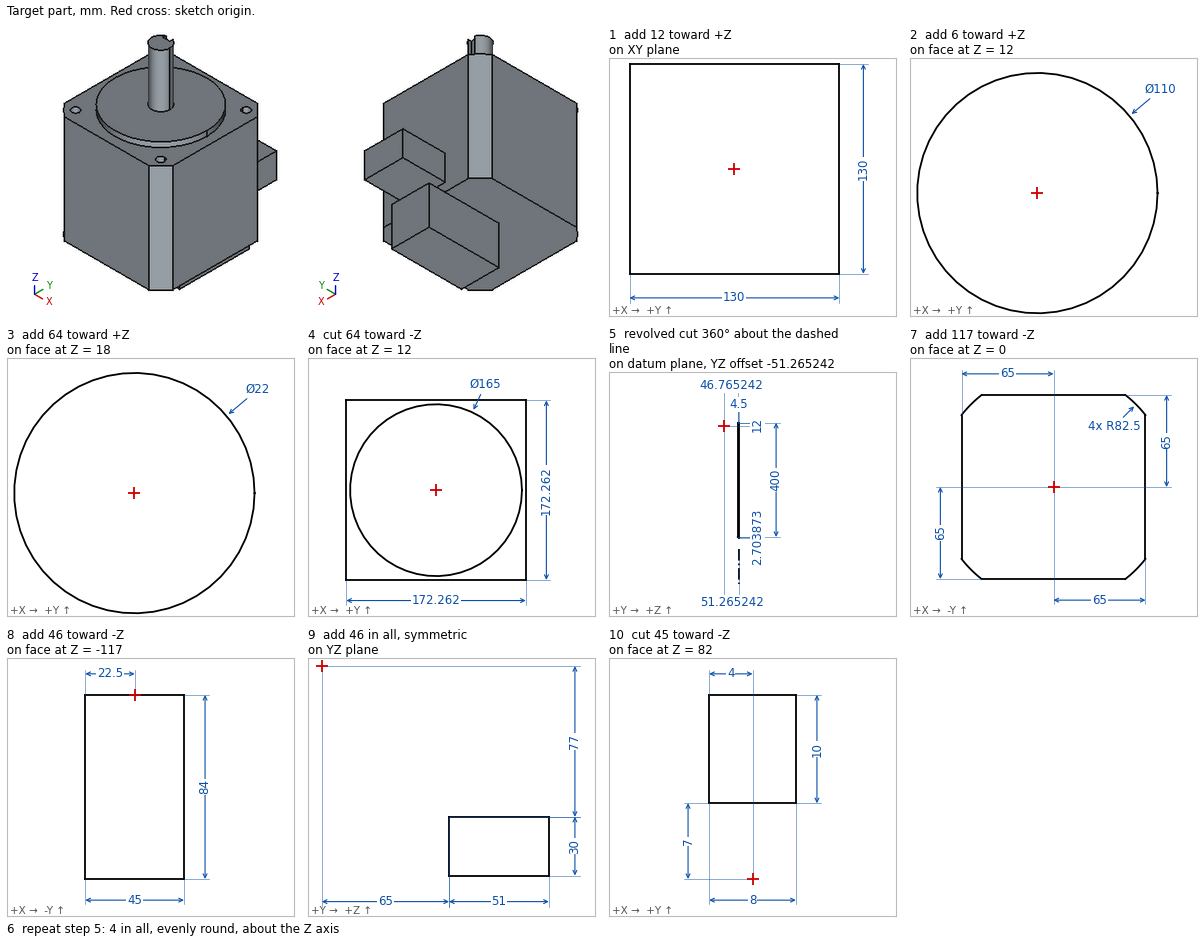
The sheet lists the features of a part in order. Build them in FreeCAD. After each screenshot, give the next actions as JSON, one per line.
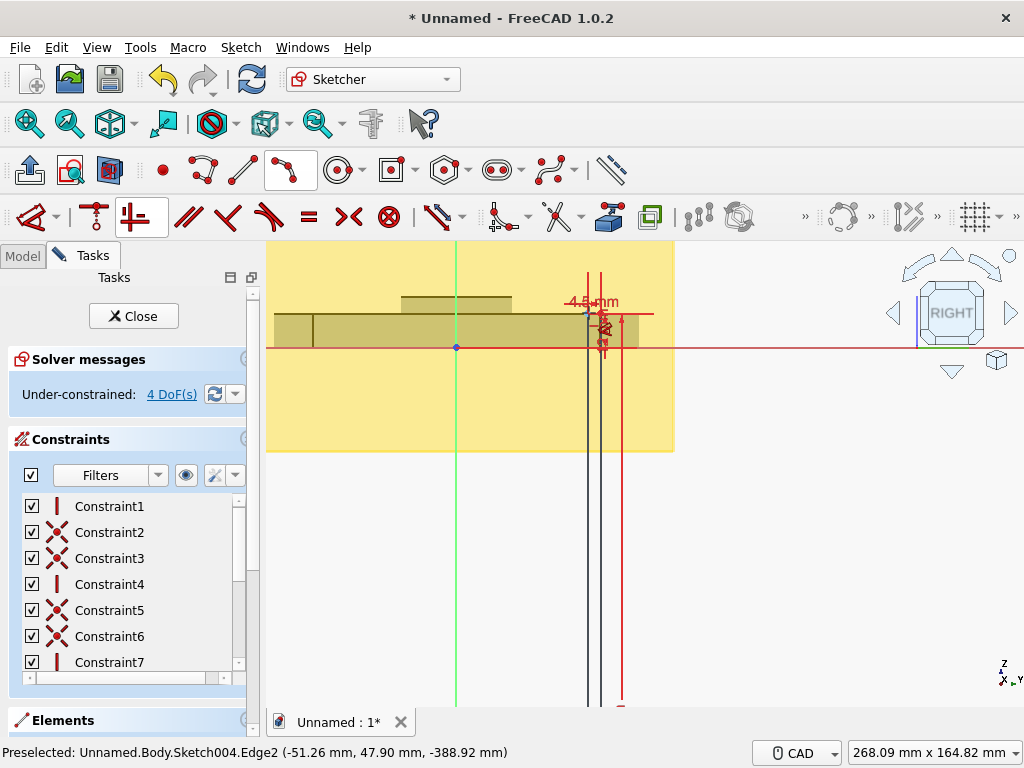
{"action": "left_click", "coordinate": [588, 314]}
{"action": "left_click", "coordinate": [522, 280]}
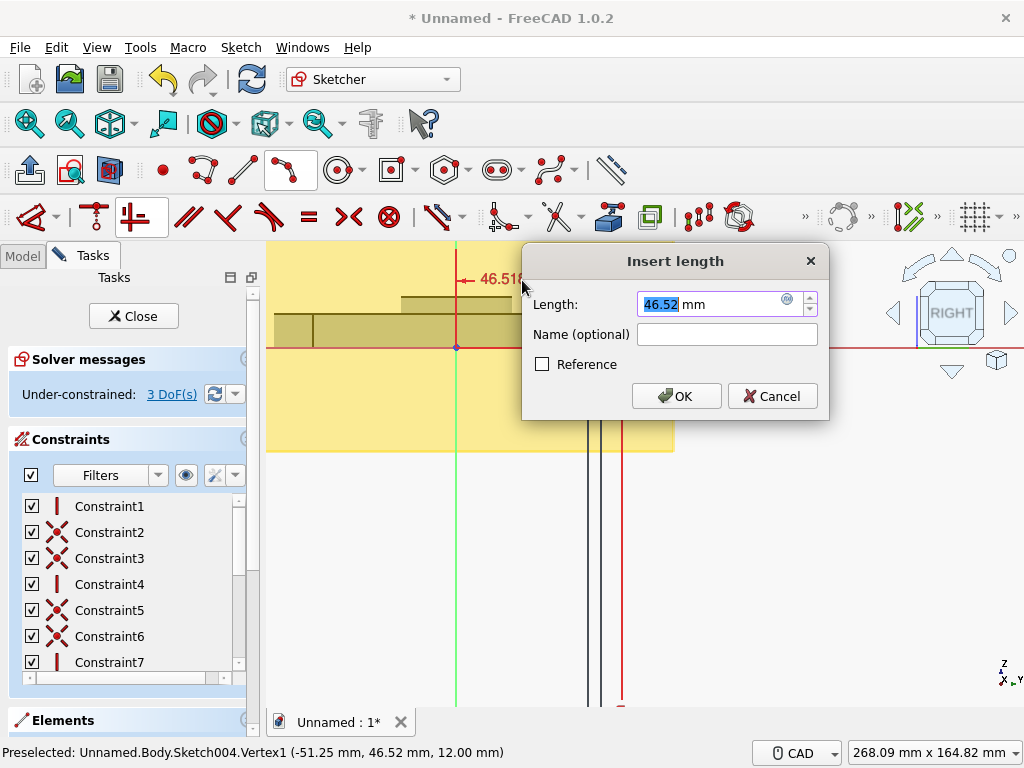
{"action": "type", "text": "46.765242"}
{"action": "key", "text": "Return"}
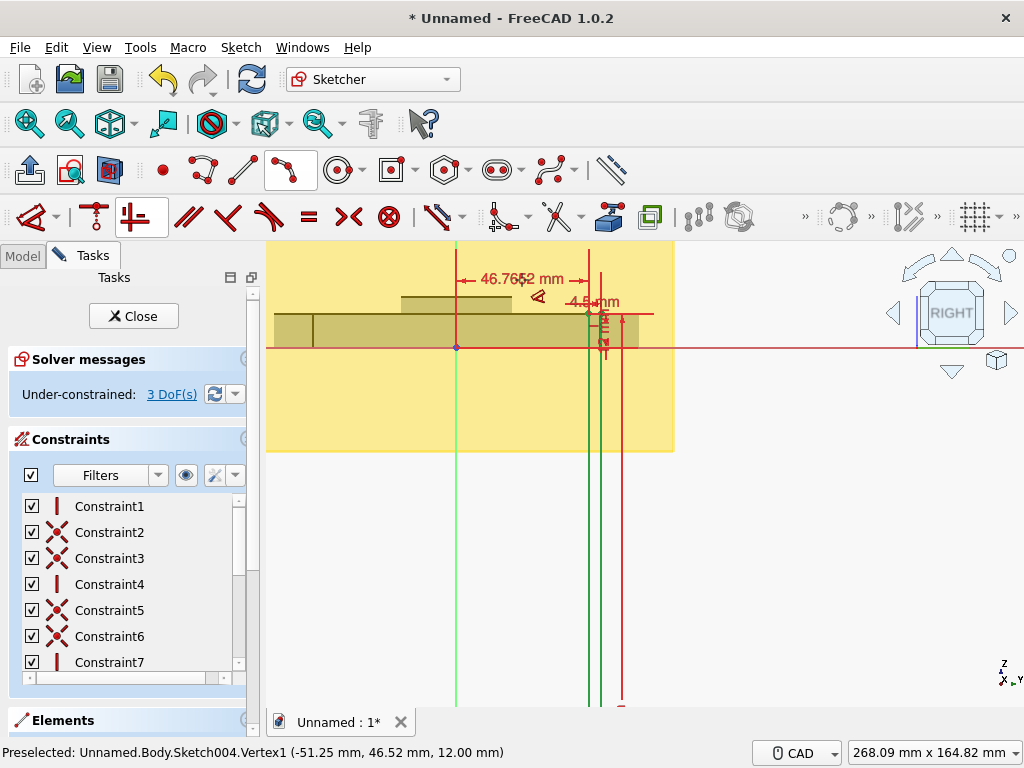
{"action": "scroll", "coordinate": [586, 348], "scroll_direction": "down", "scroll_amount": 9}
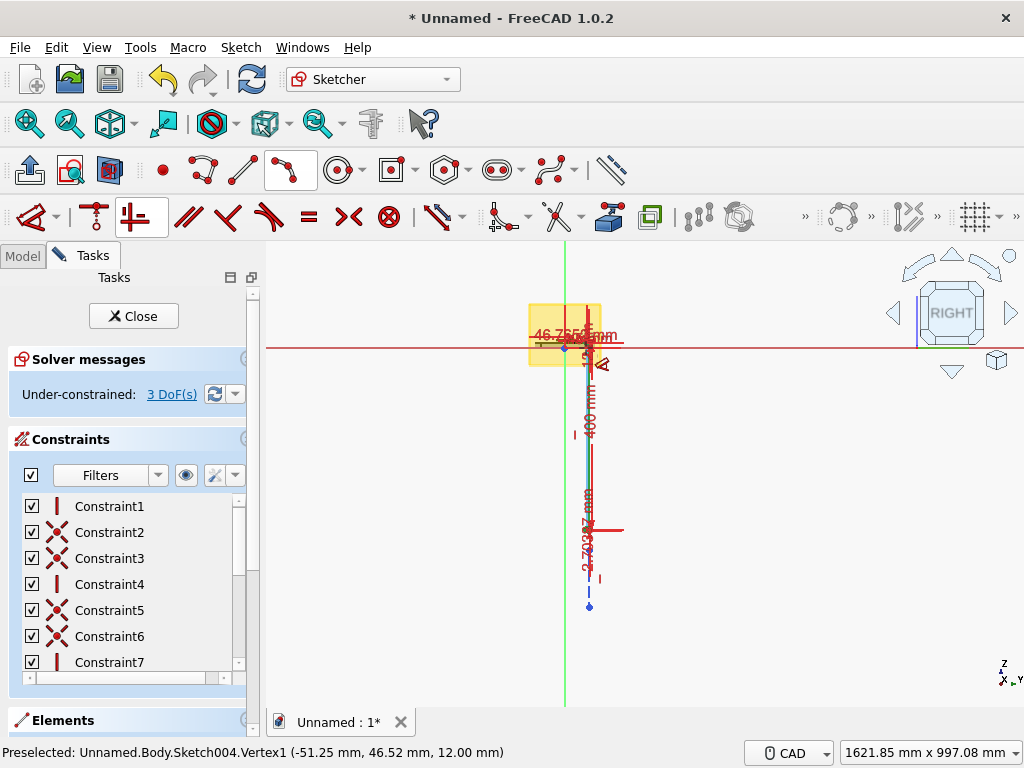
{"action": "scroll", "coordinate": [589, 550], "scroll_direction": "up", "scroll_amount": 3}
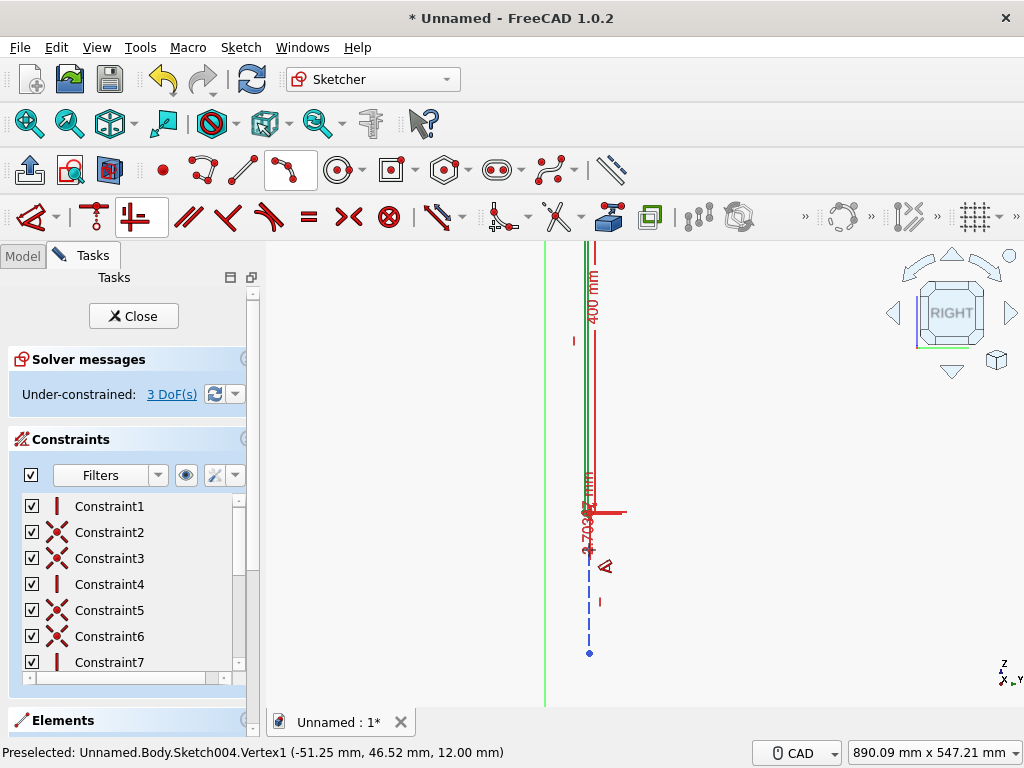
{"action": "left_click", "coordinate": [589, 550]}
{"action": "left_click", "coordinate": [567, 584]}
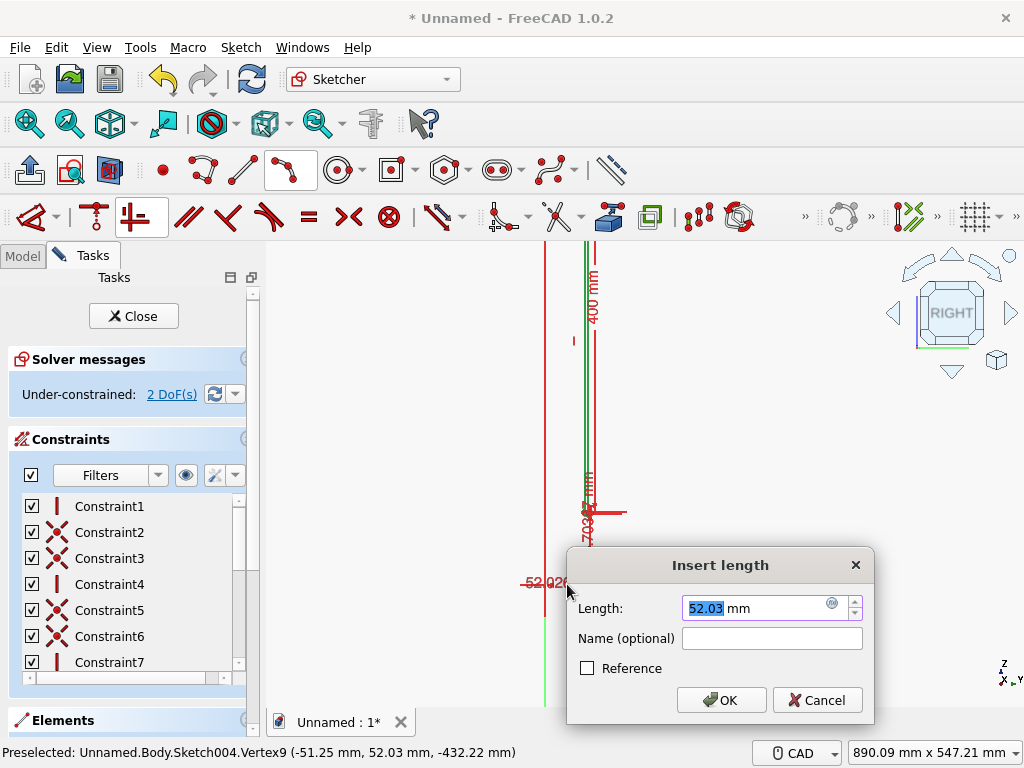
{"action": "type", "text": "51.265242"}
{"action": "key", "text": "Return"}
{"action": "key", "text": "Escape"}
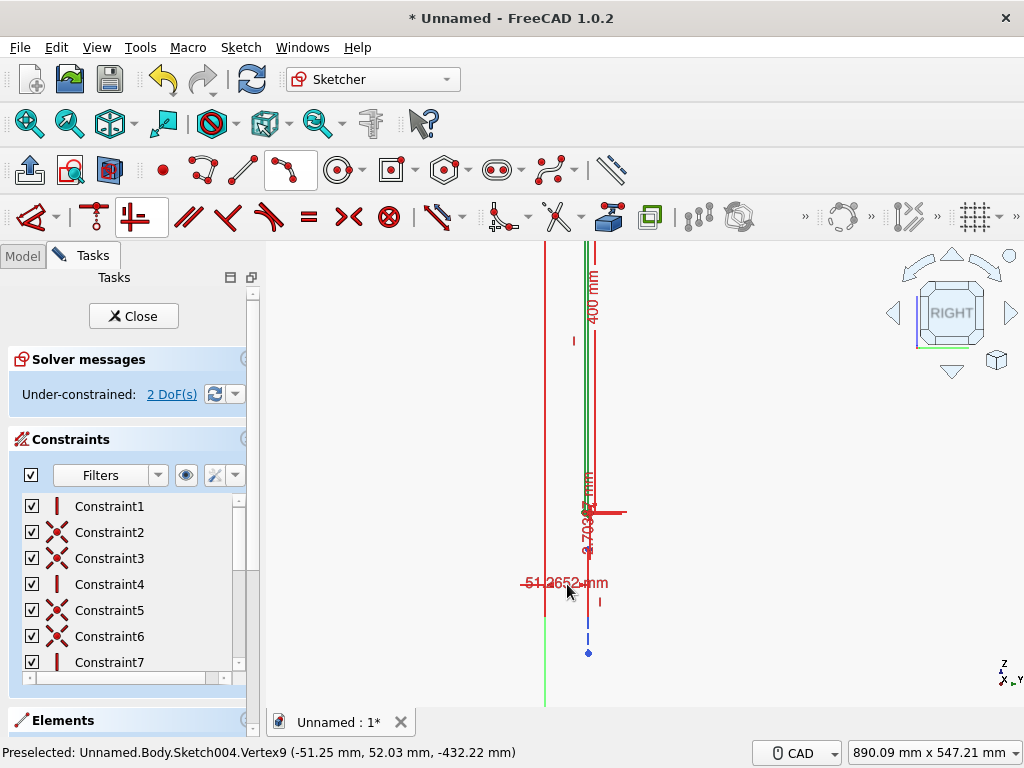
{"action": "left_click", "coordinate": [134, 316]}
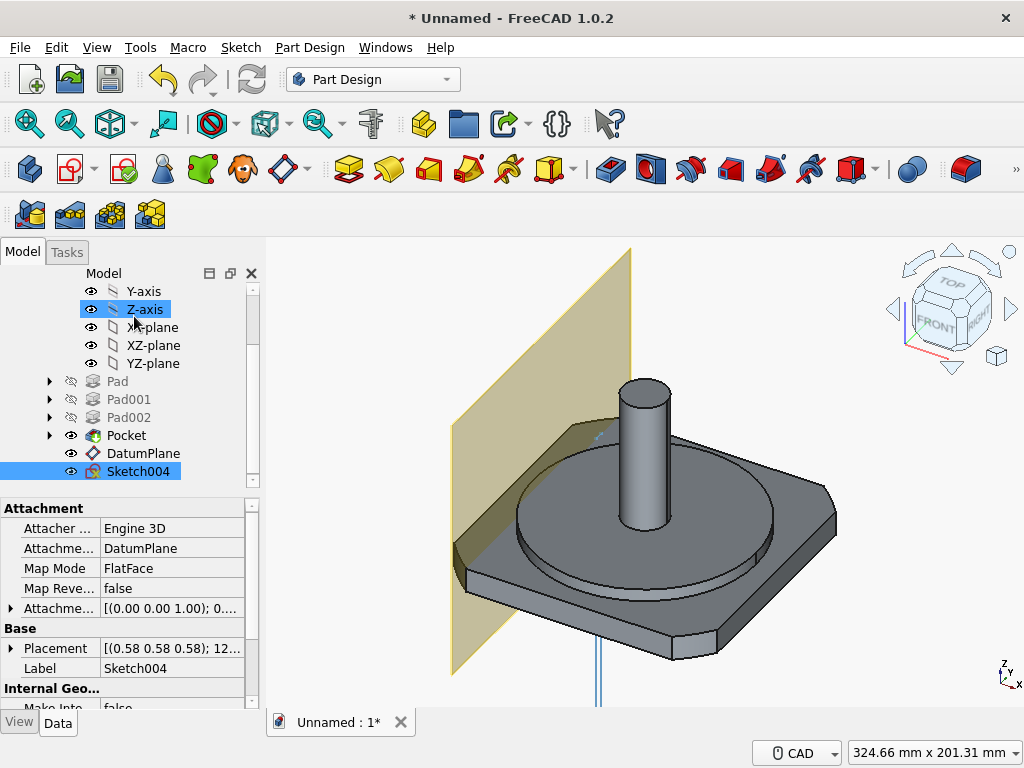
{"action": "left_click", "coordinate": [692, 170]}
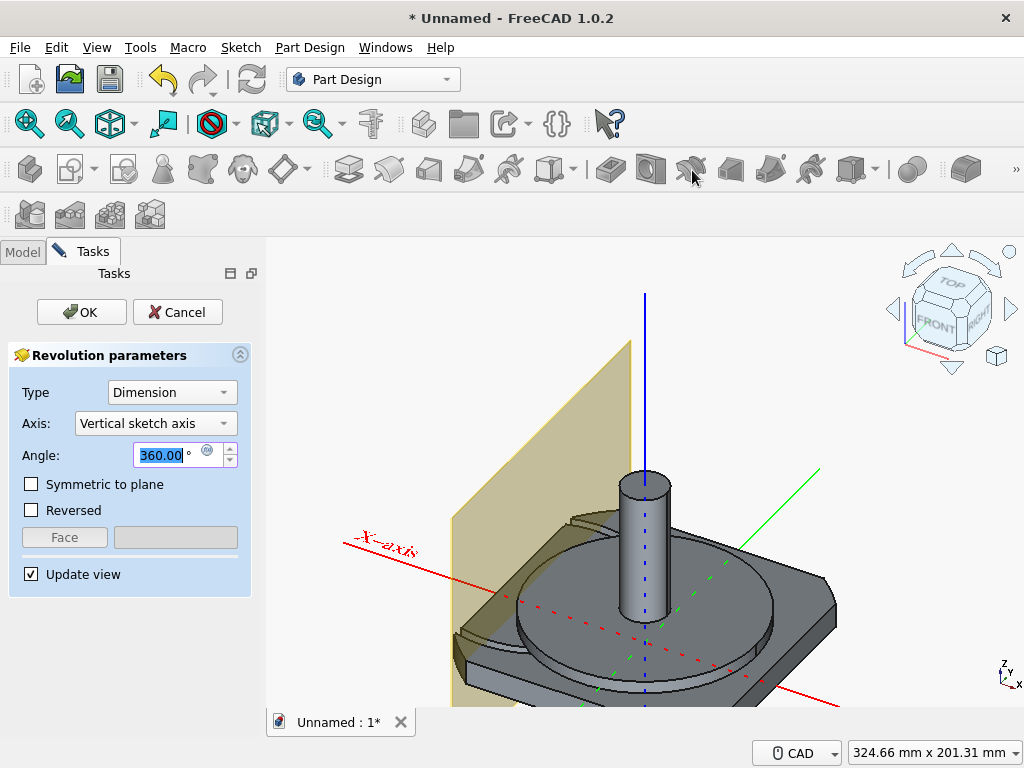
{"action": "left_click", "coordinate": [156, 424]}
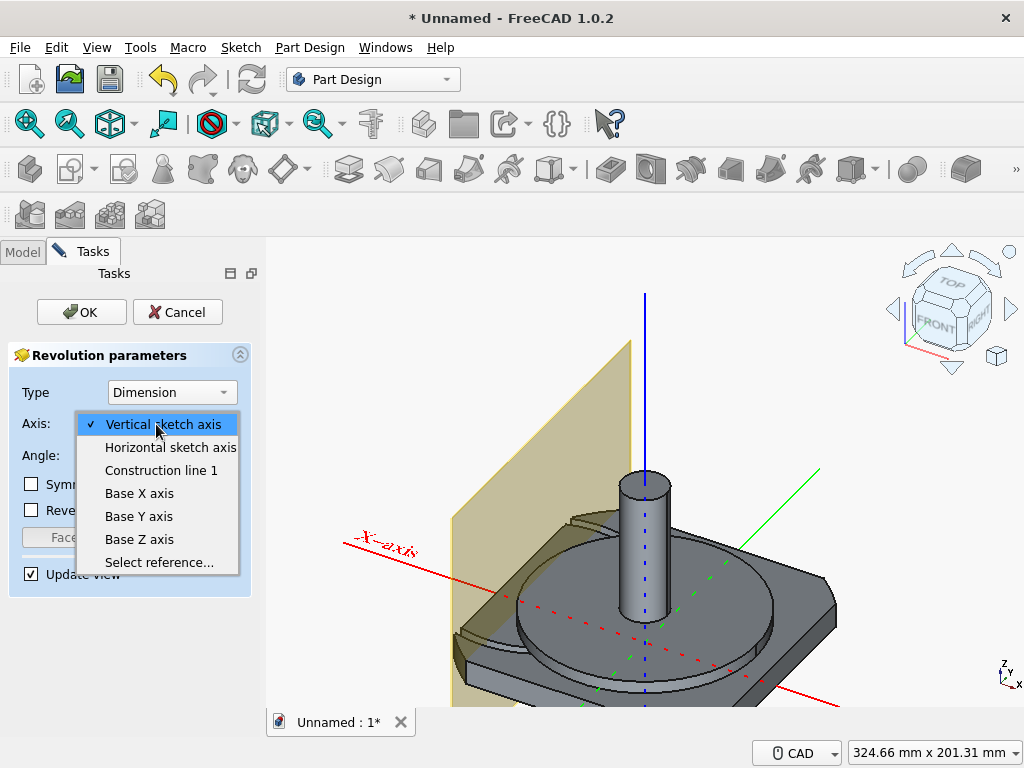
{"action": "left_click", "coordinate": [156, 470]}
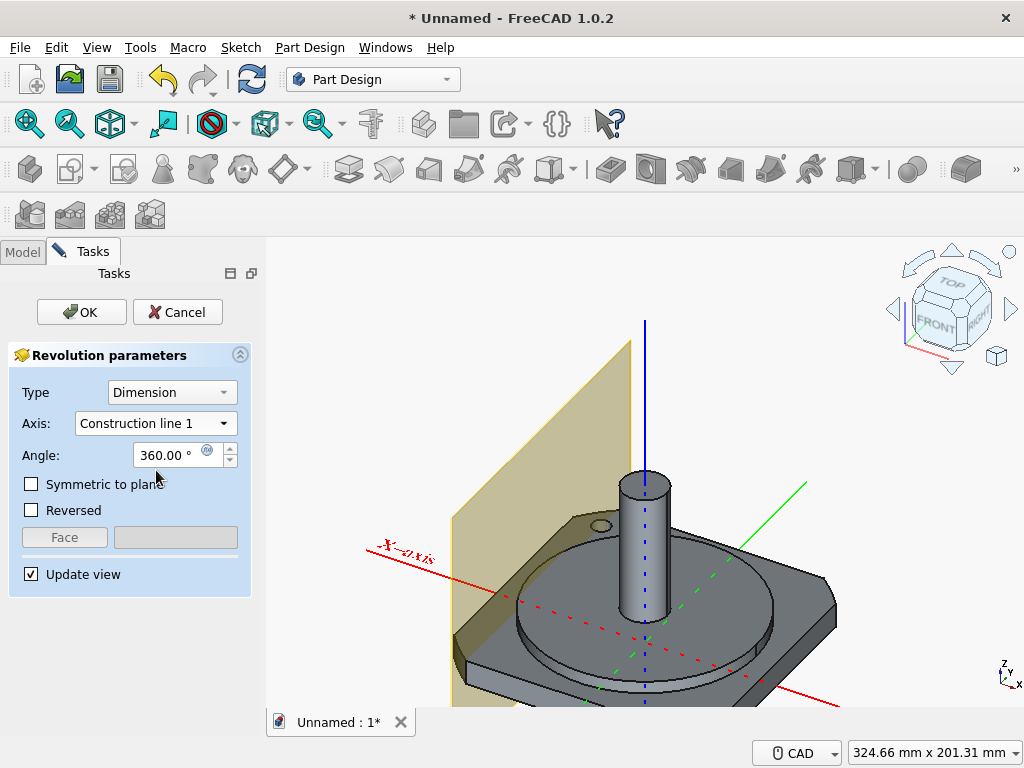
{"action": "left_click", "coordinate": [82, 312]}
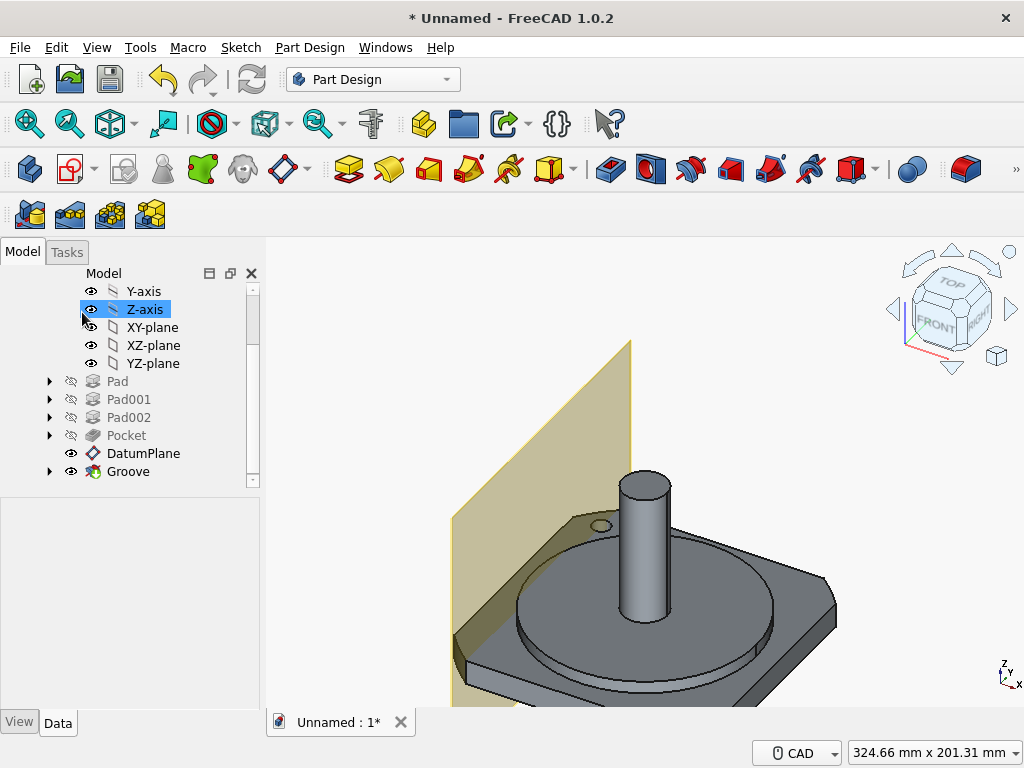
{"action": "left_click", "coordinate": [116, 453]}
{"action": "key", "text": "space"}